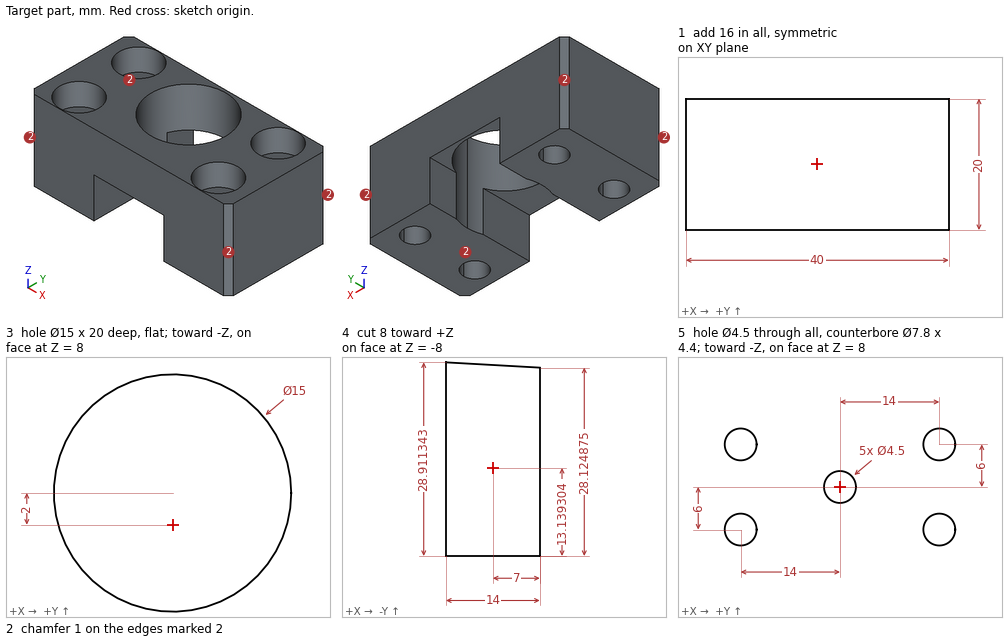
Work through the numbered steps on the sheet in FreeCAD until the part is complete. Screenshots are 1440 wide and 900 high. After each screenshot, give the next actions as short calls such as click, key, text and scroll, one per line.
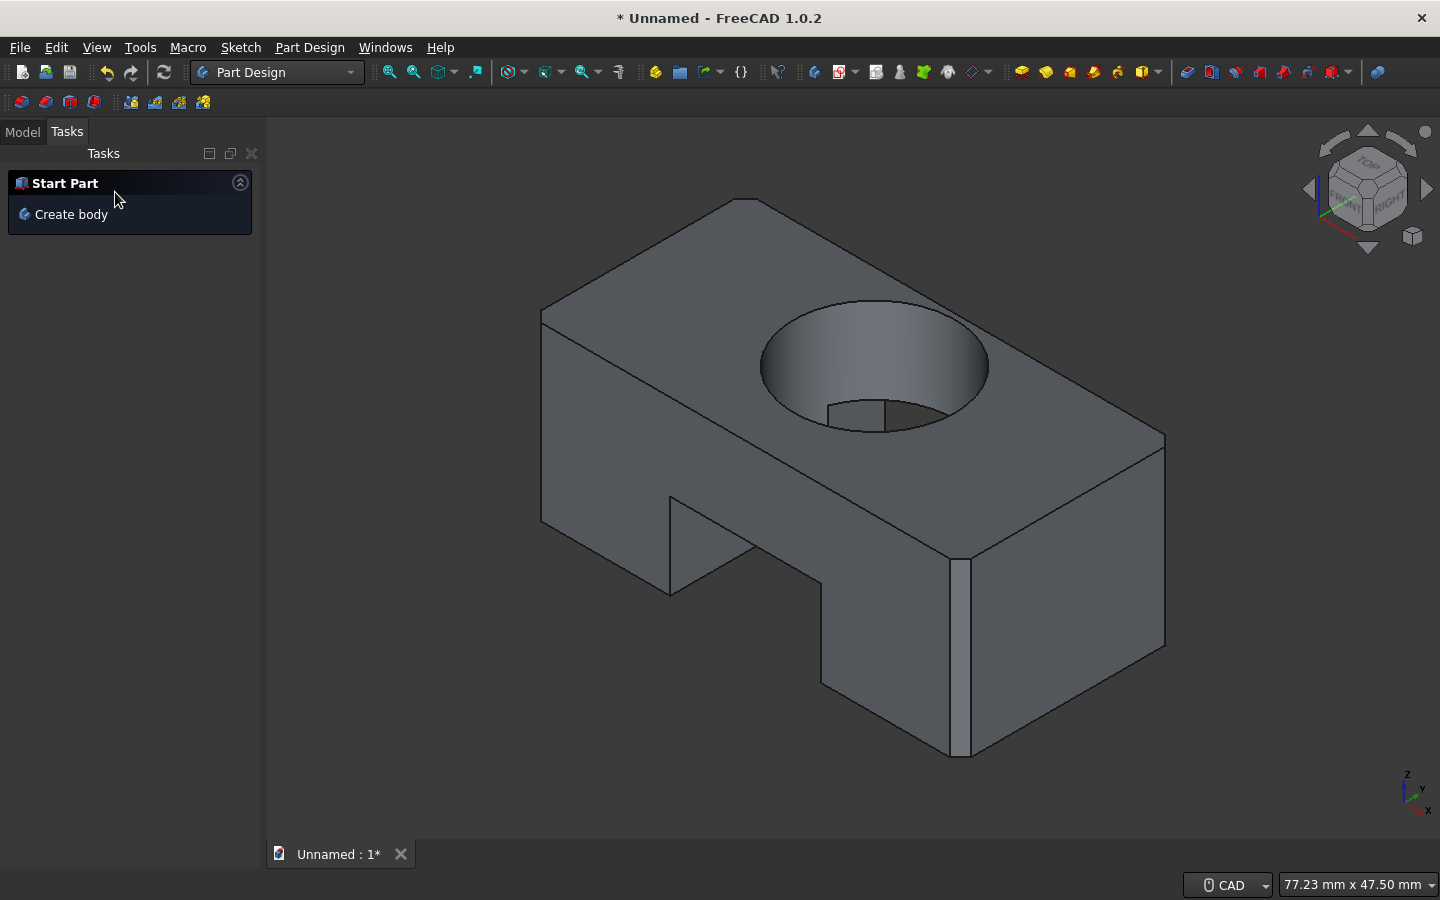
click(699, 325)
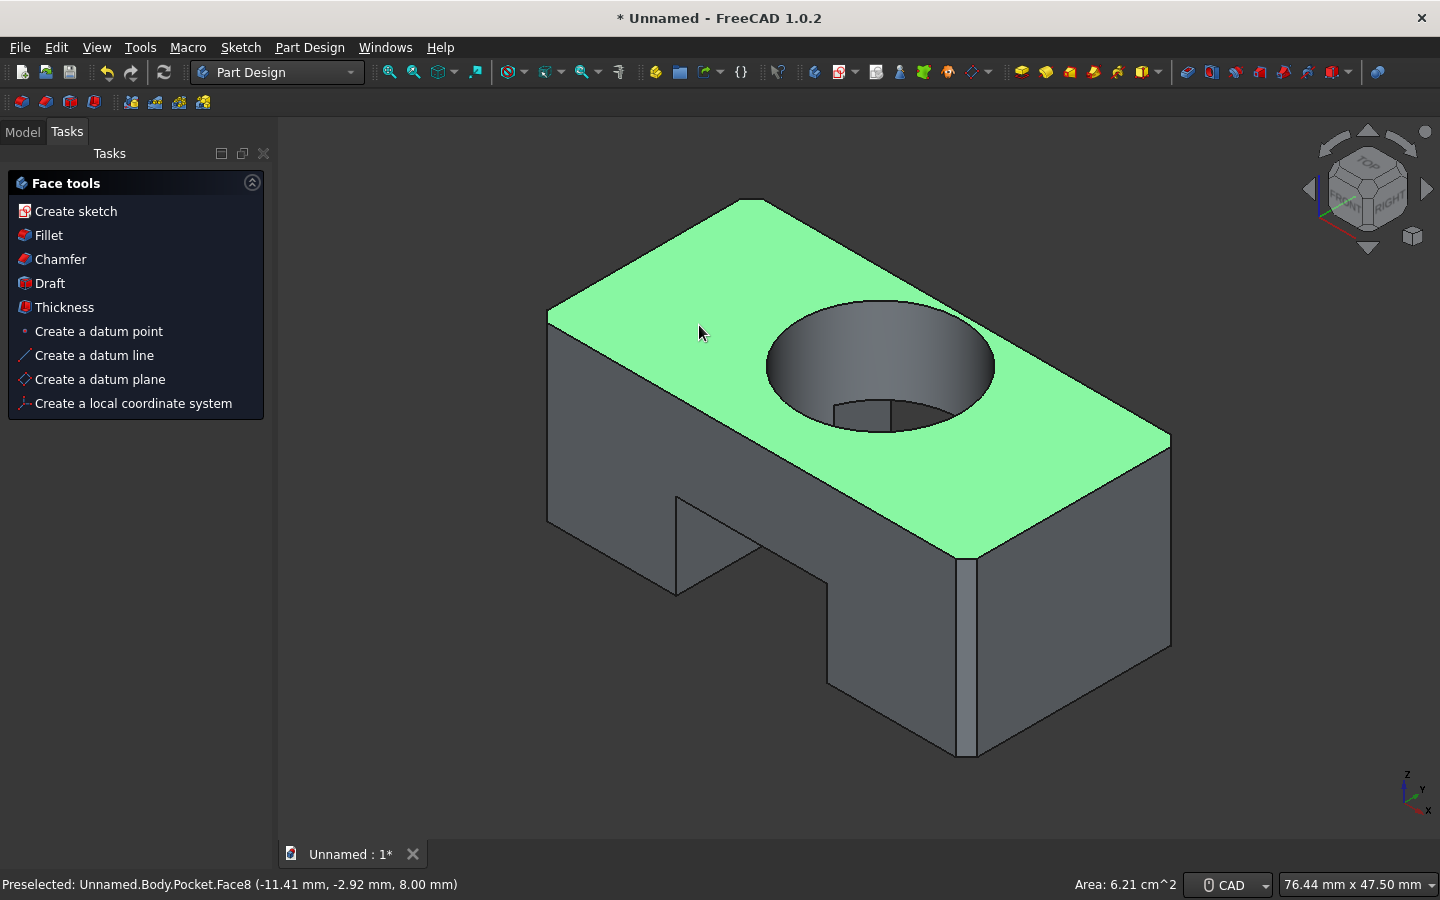
click(840, 72)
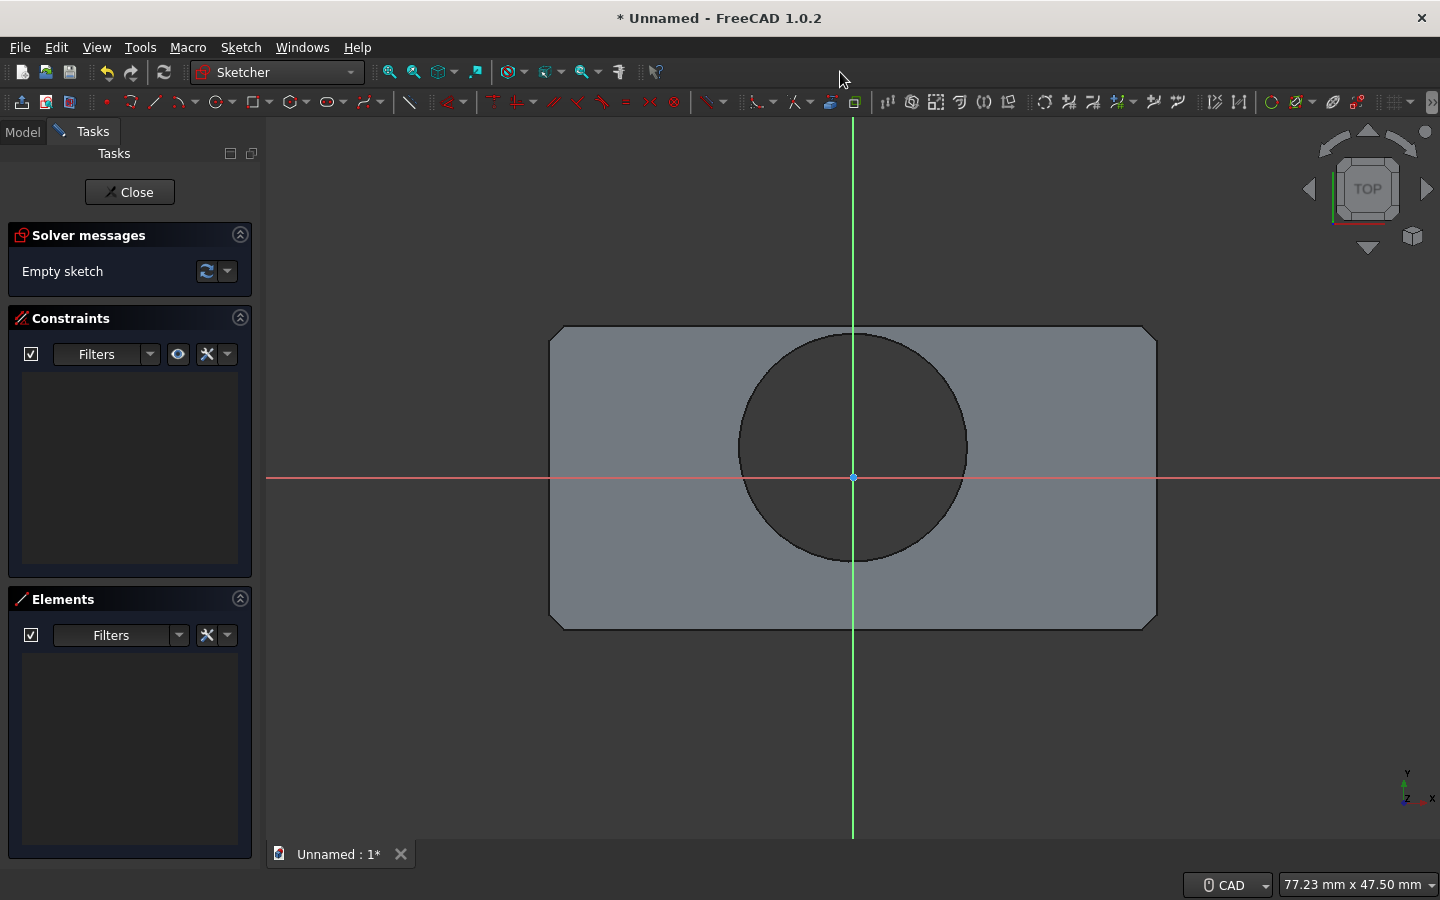
scroll(992, 478, up, 2)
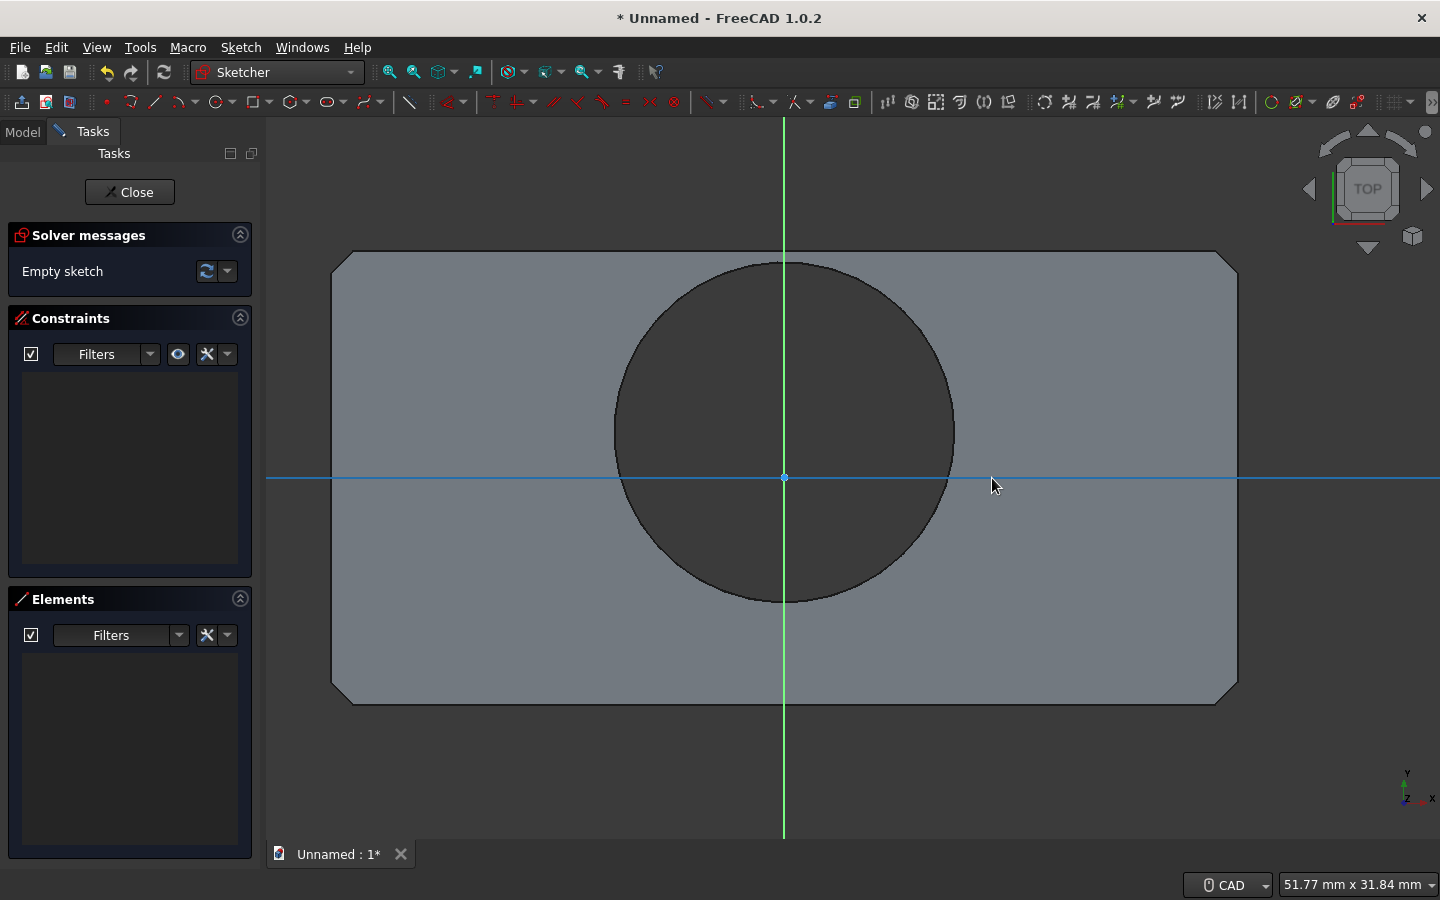
key(g)
key(c)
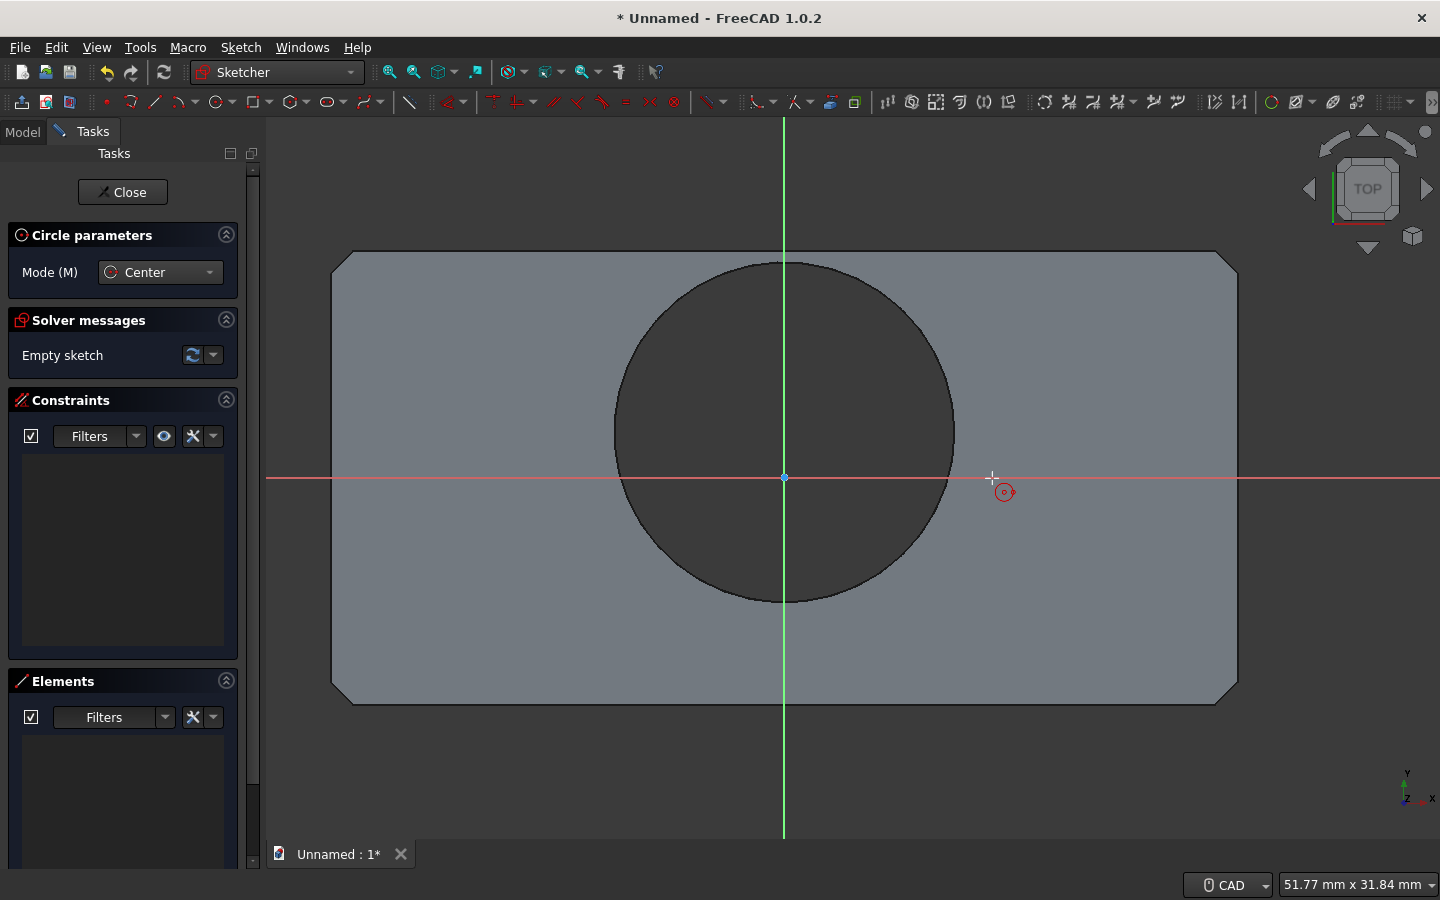
click(784, 478)
click(820, 442)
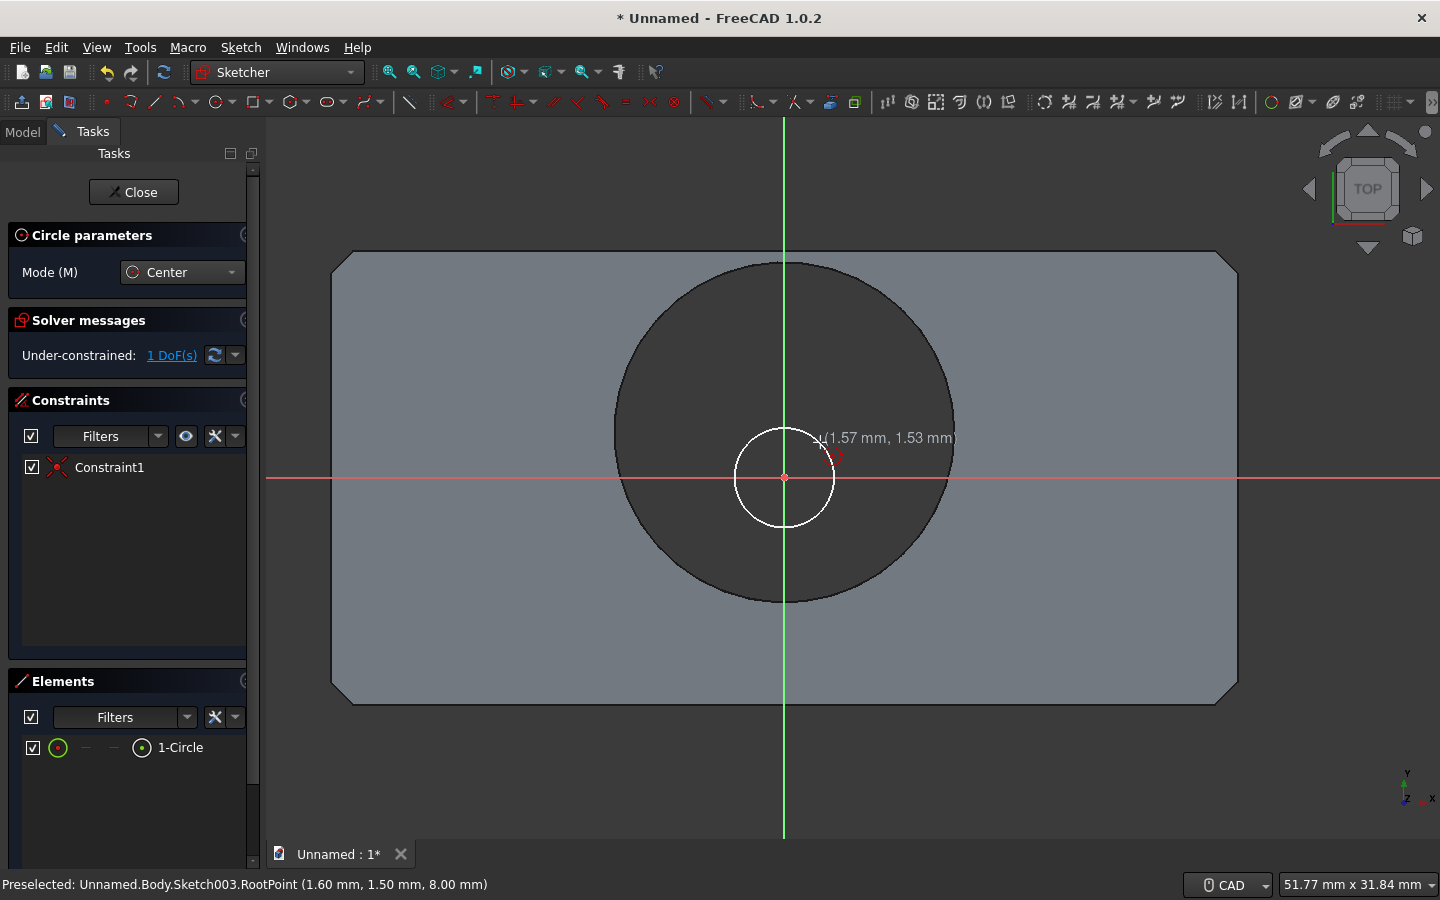
click(1102, 342)
click(1138, 306)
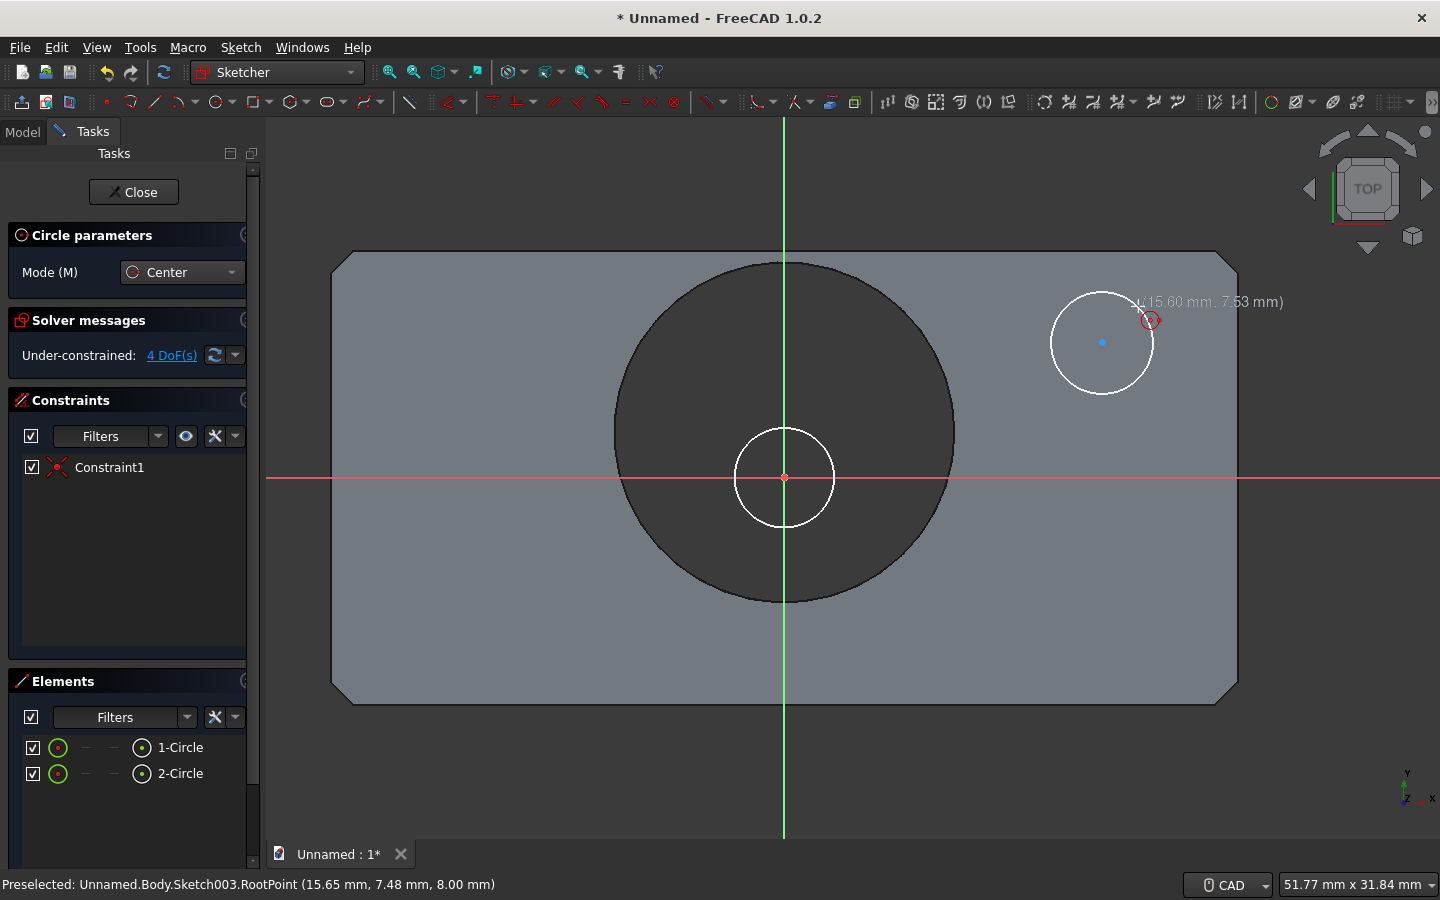
click(467, 614)
click(503, 578)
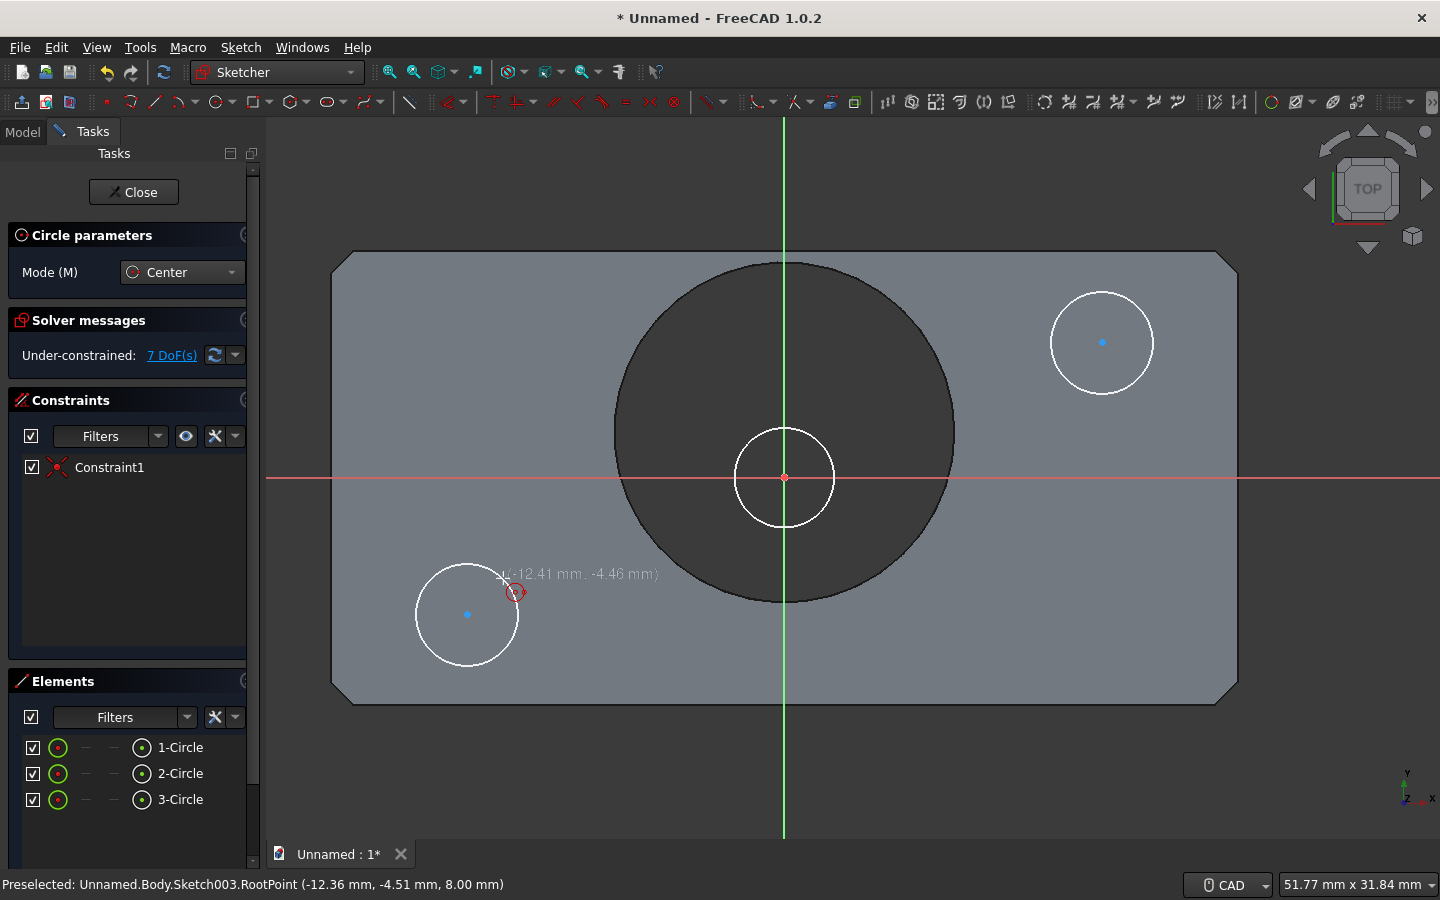
click(467, 342)
click(503, 306)